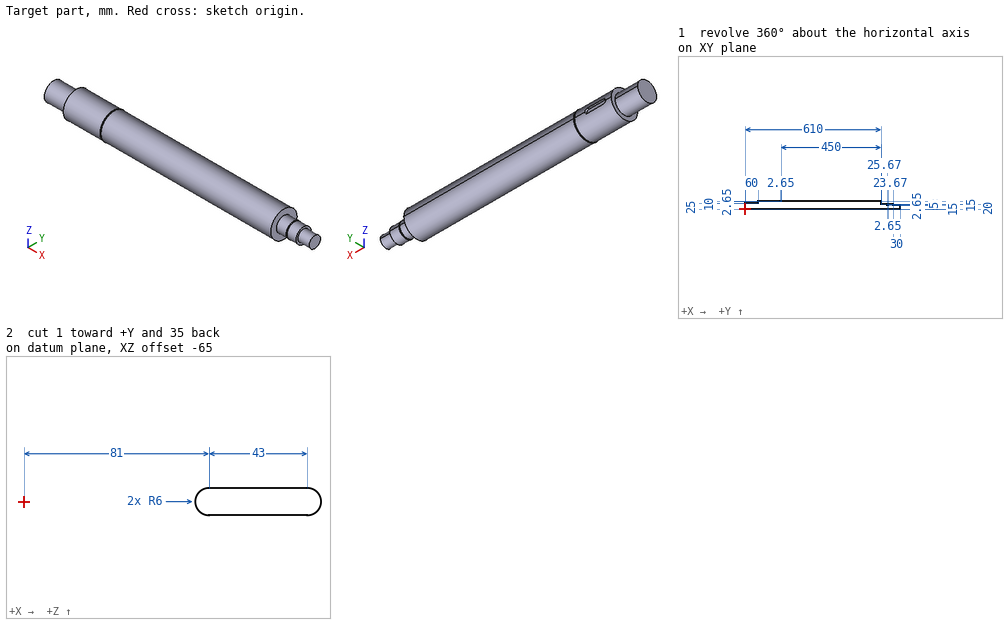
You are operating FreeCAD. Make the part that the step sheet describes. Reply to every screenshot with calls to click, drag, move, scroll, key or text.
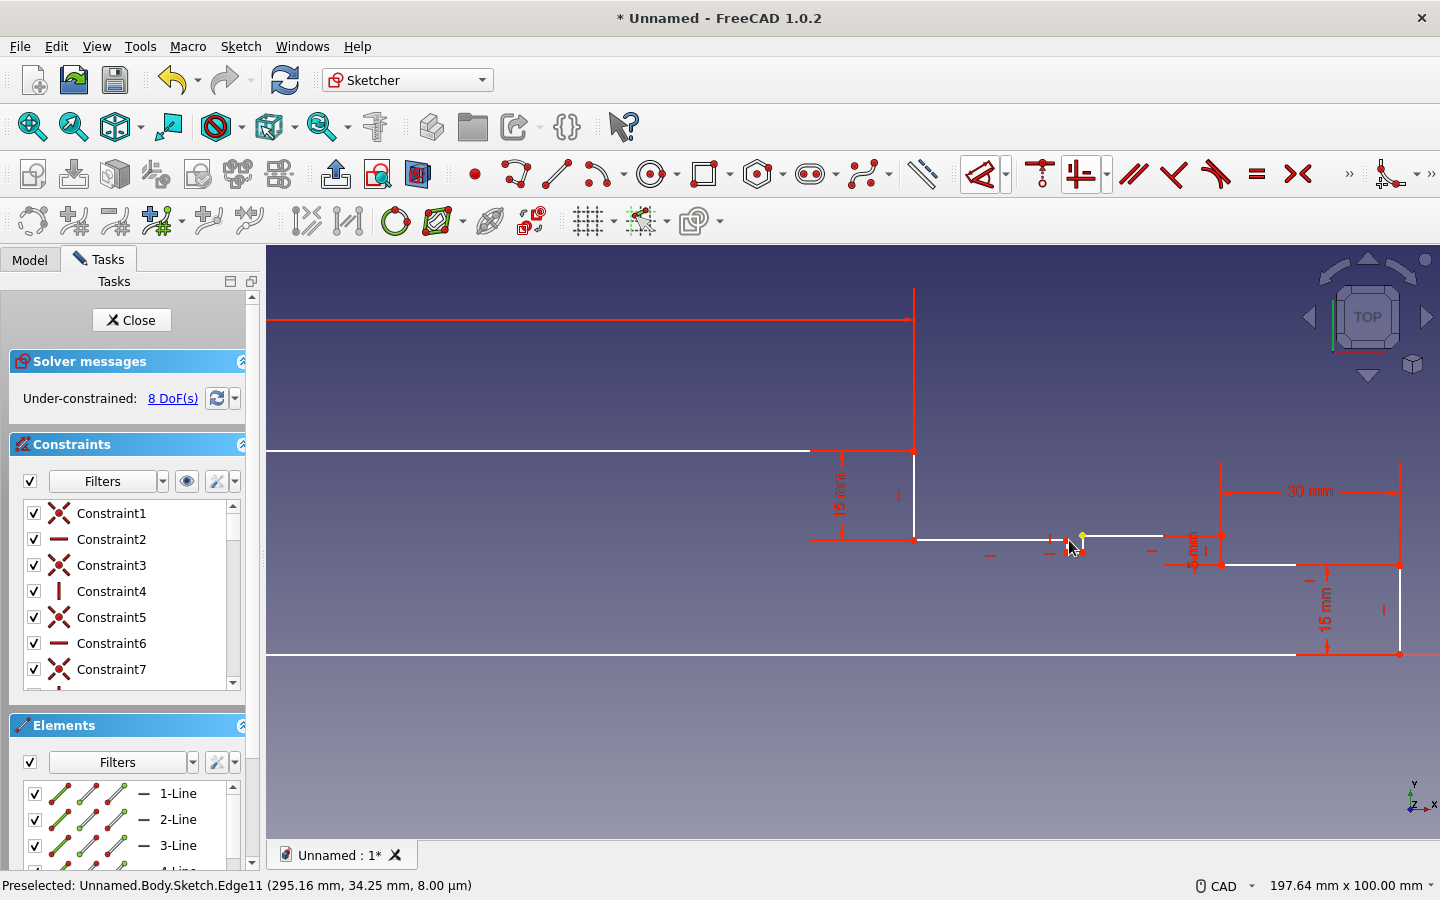
click(1067, 540)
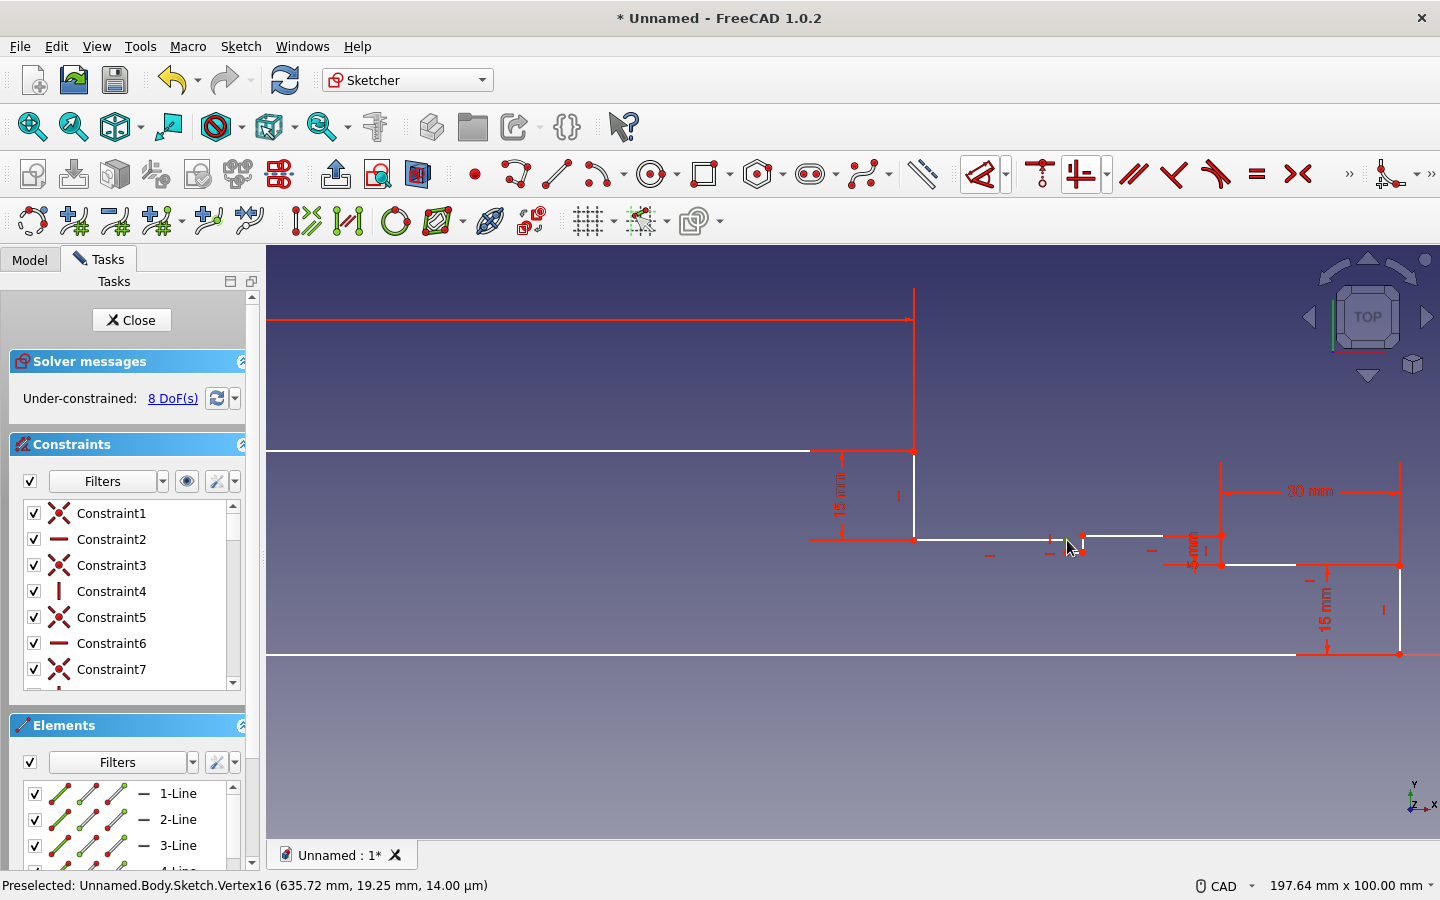
key(i)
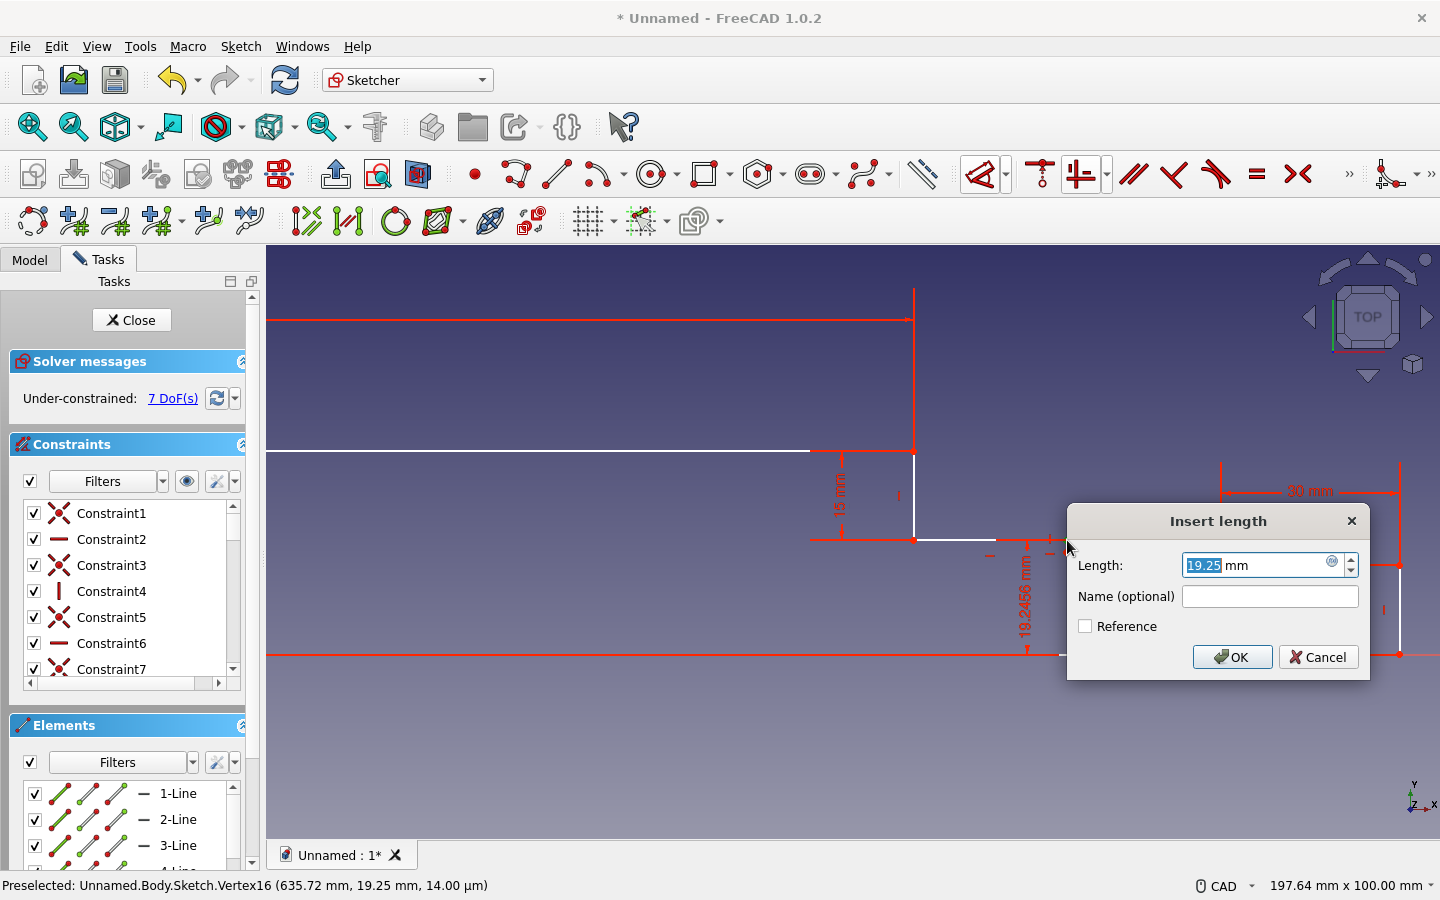
text(20)
key(Return)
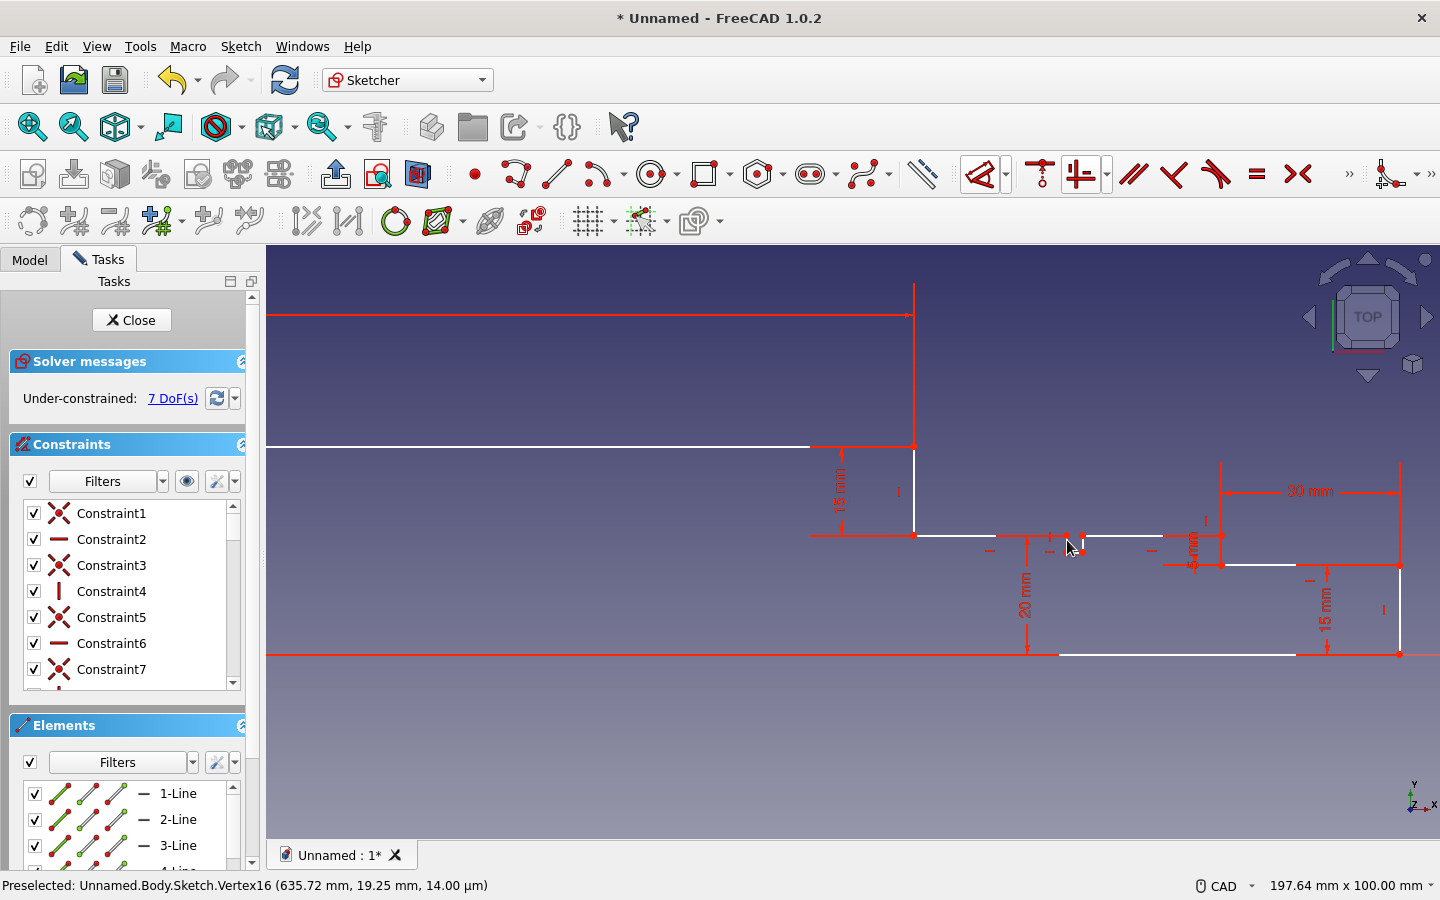
scroll(1083, 544, up, 5)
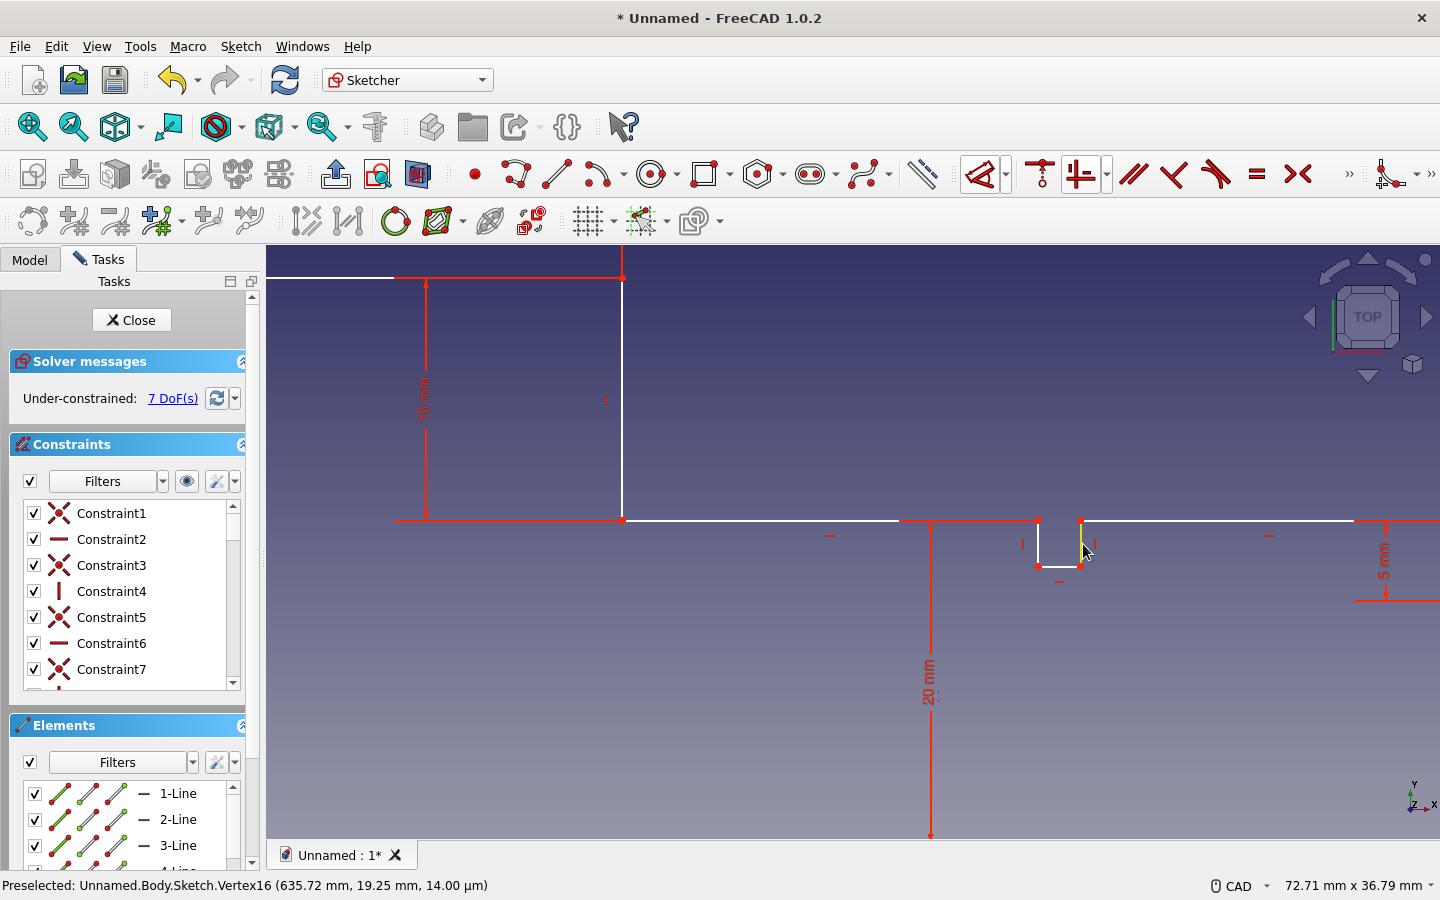
click(1081, 544)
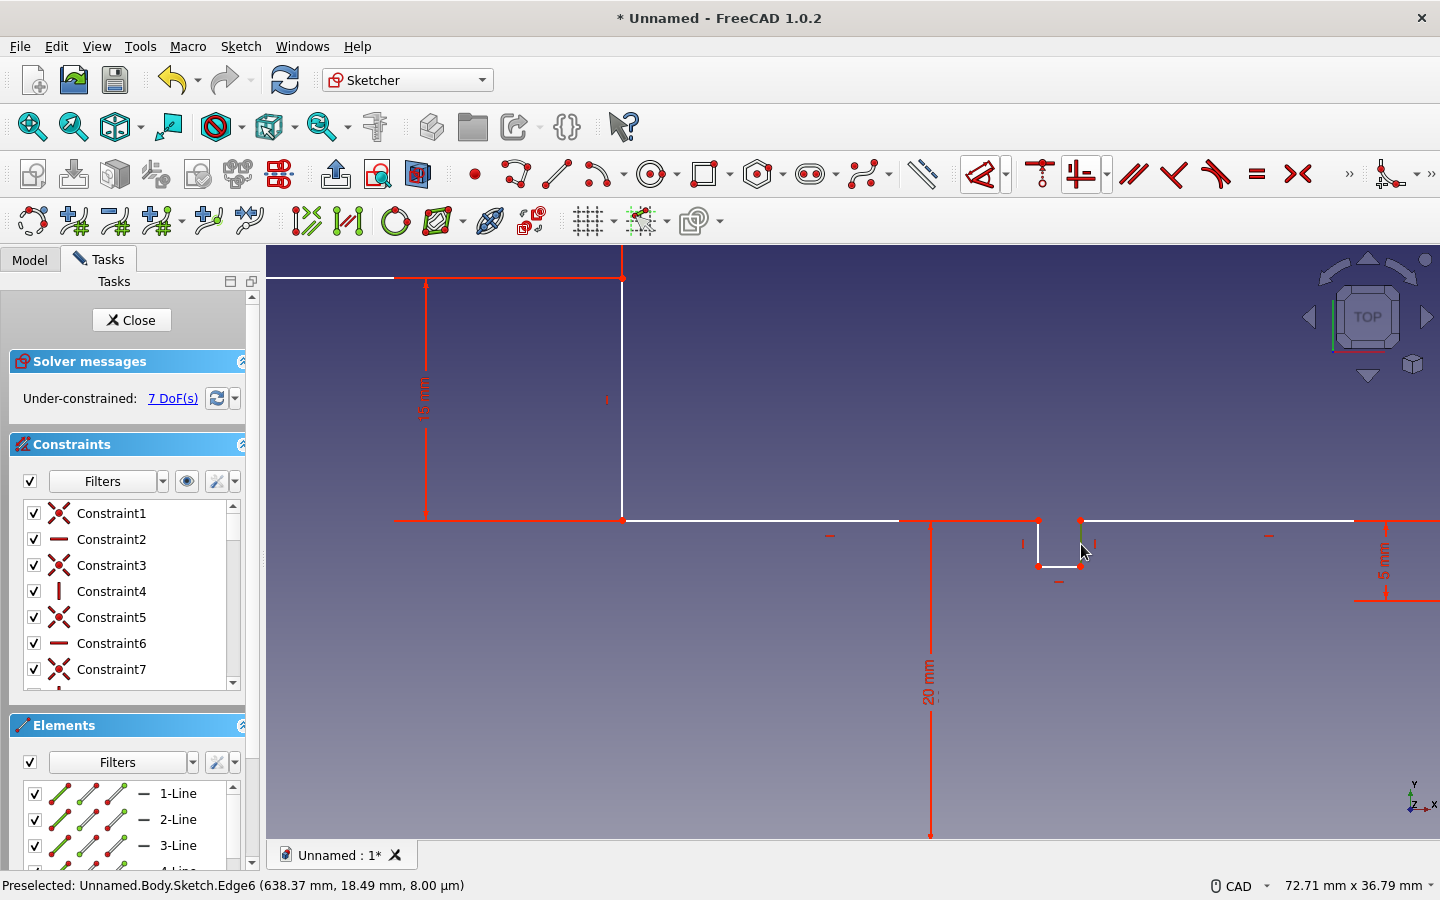
click(1006, 174)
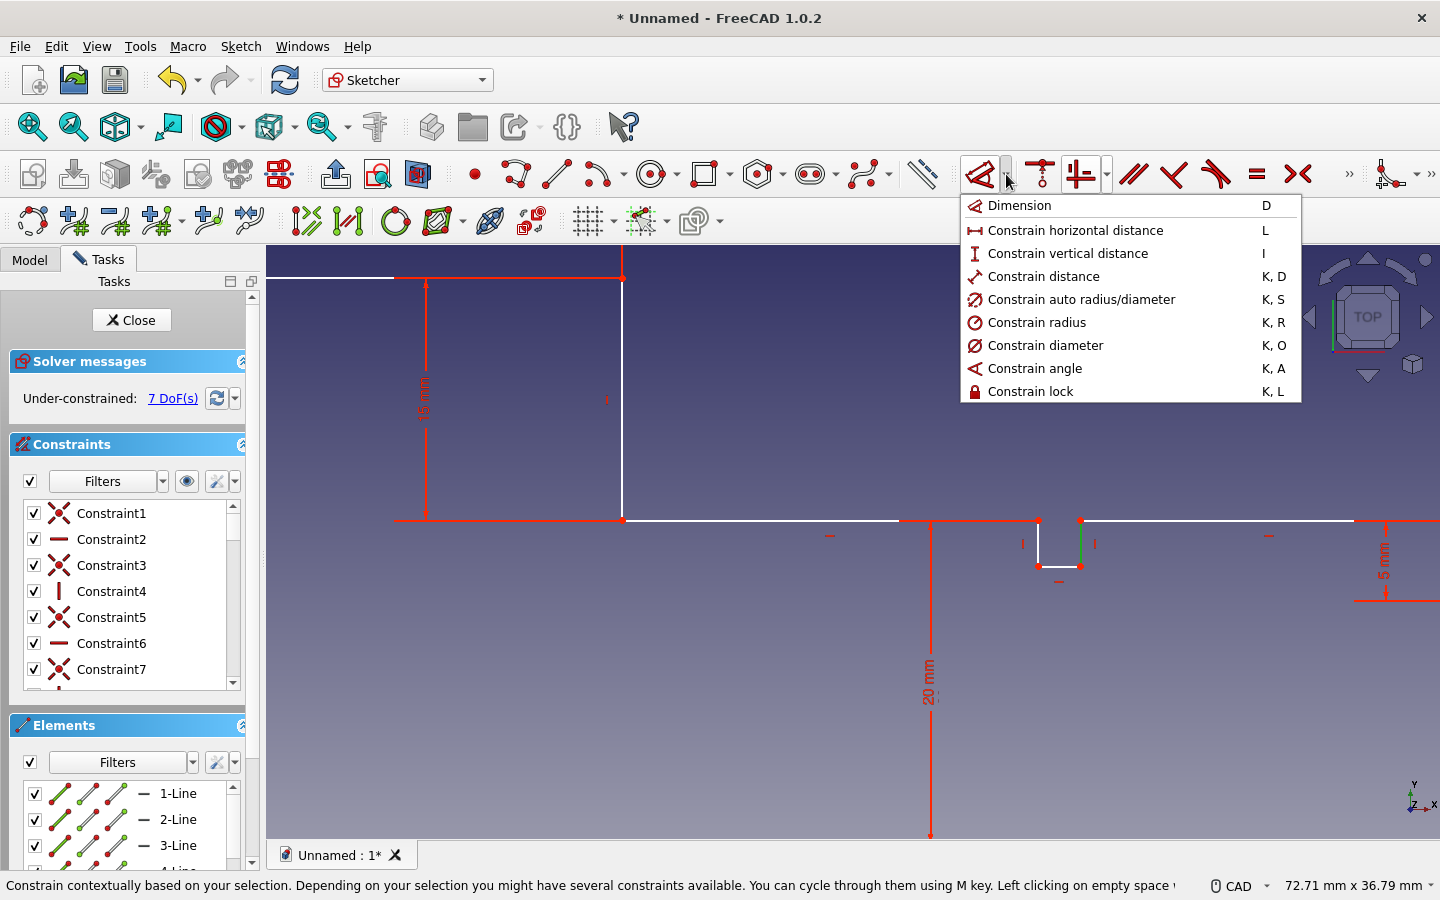
click(1131, 254)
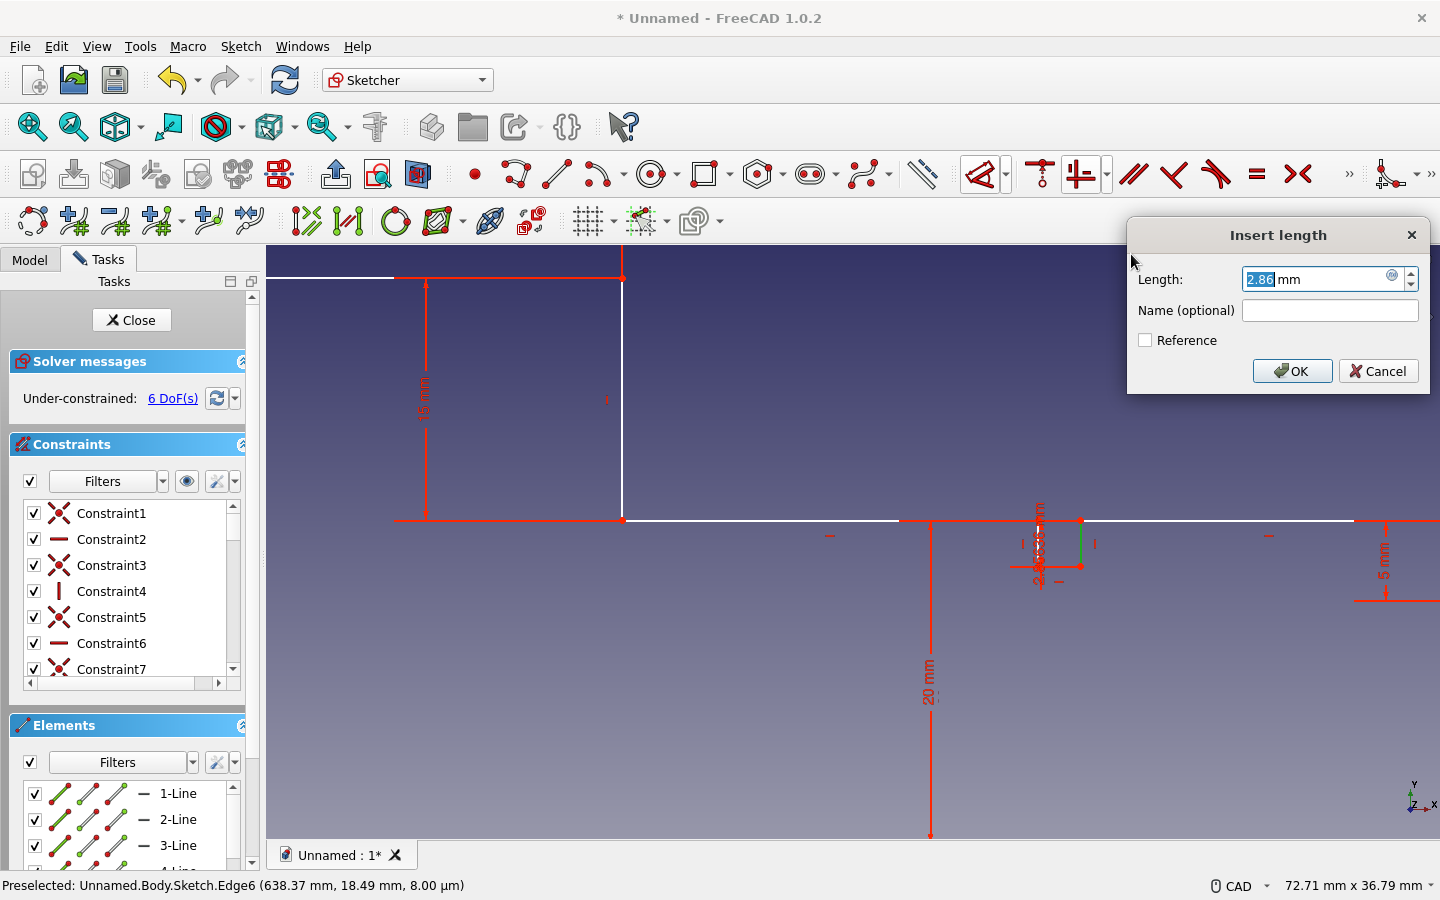
text(2.65)
key(Return)